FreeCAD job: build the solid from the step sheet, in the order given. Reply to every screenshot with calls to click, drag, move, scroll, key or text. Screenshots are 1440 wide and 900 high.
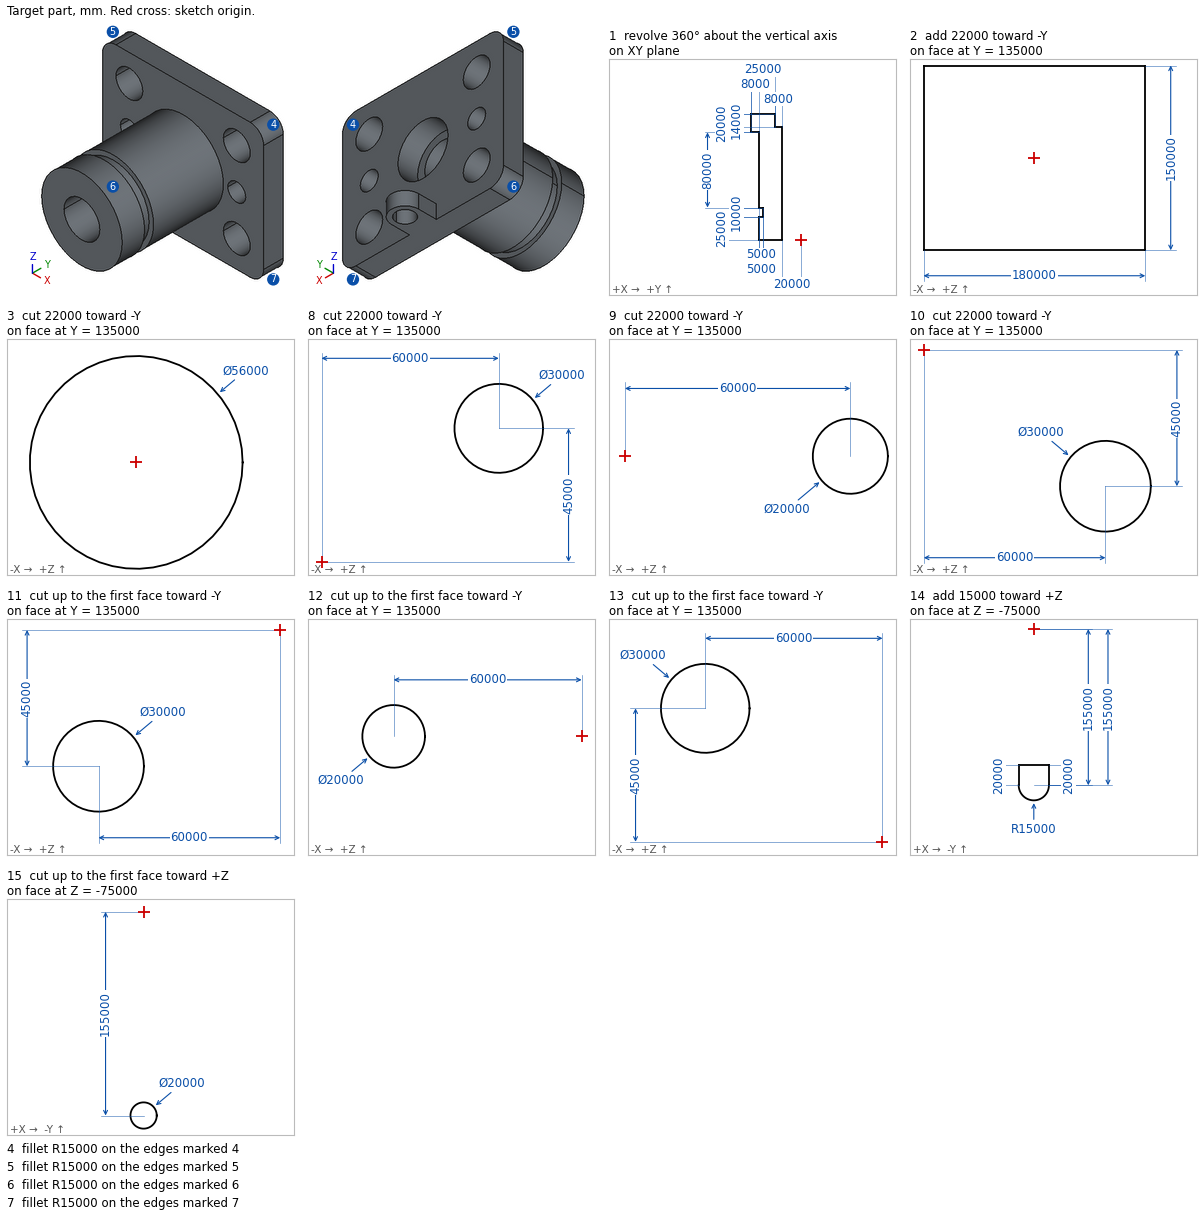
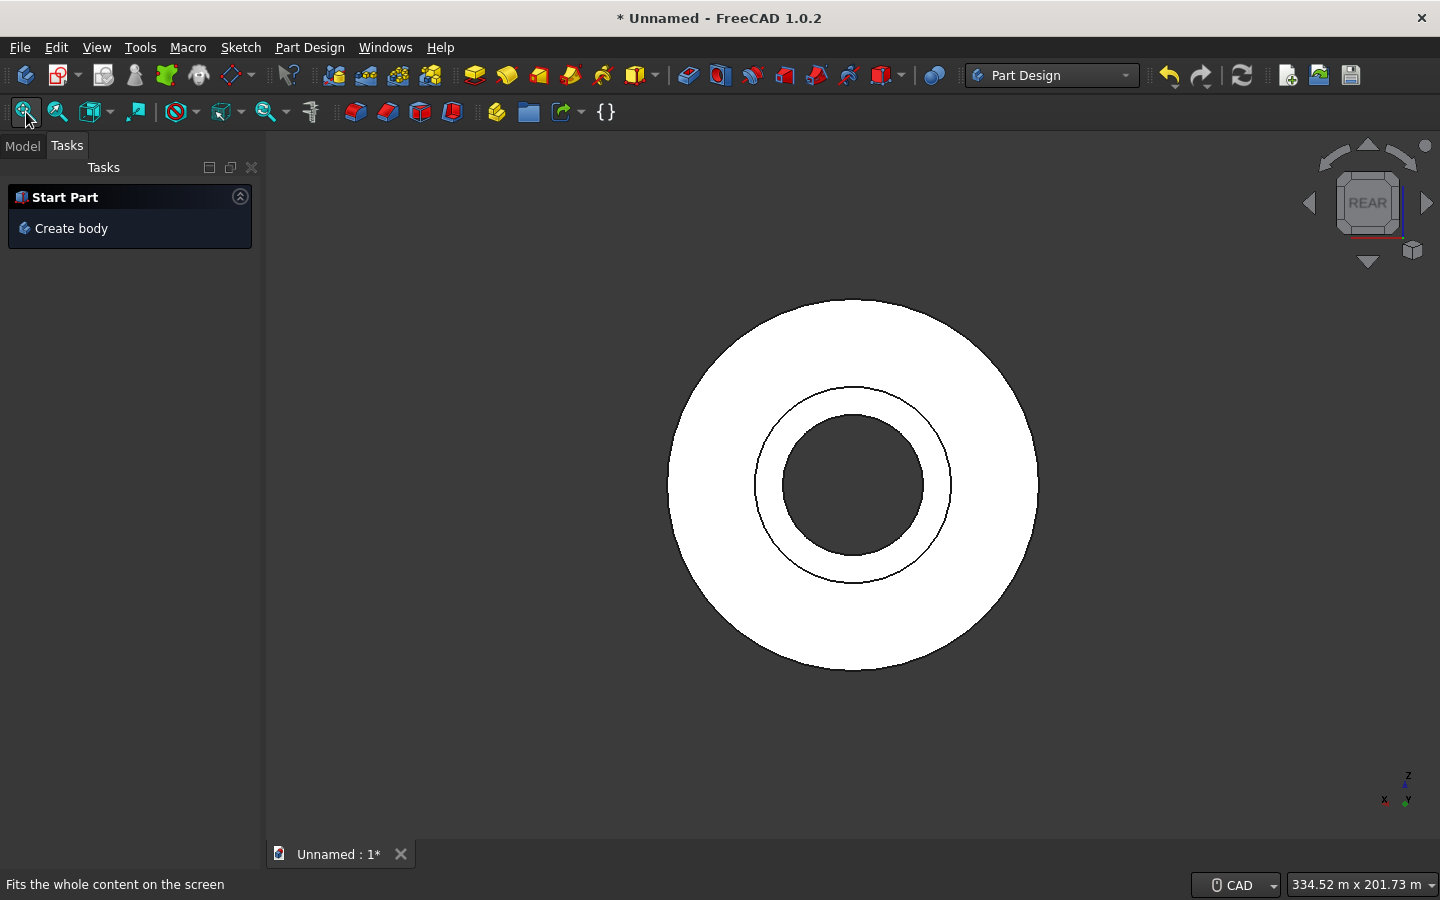
click(747, 590)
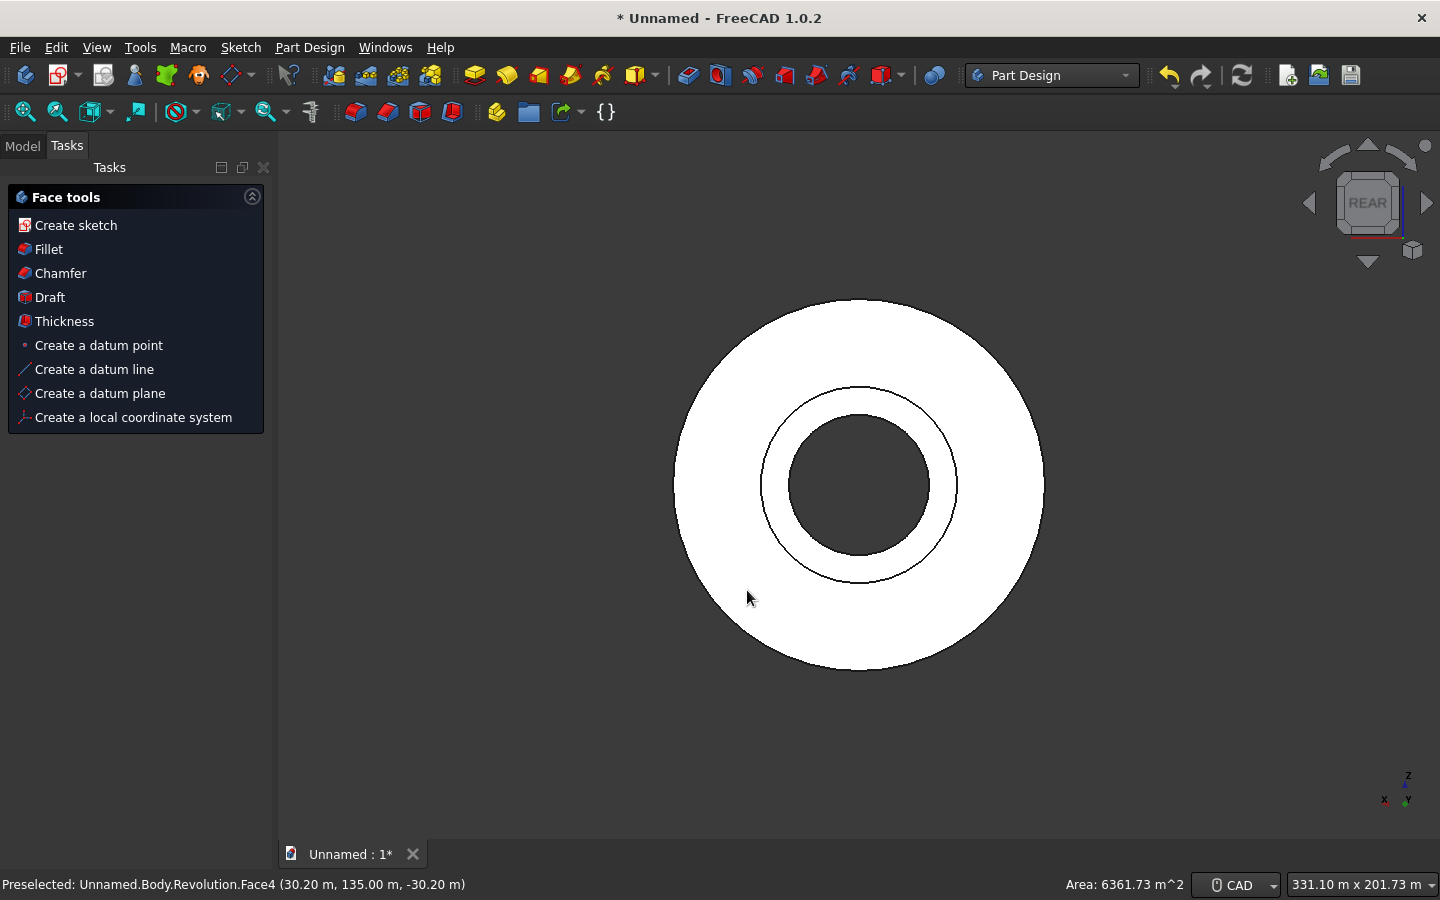
click(58, 76)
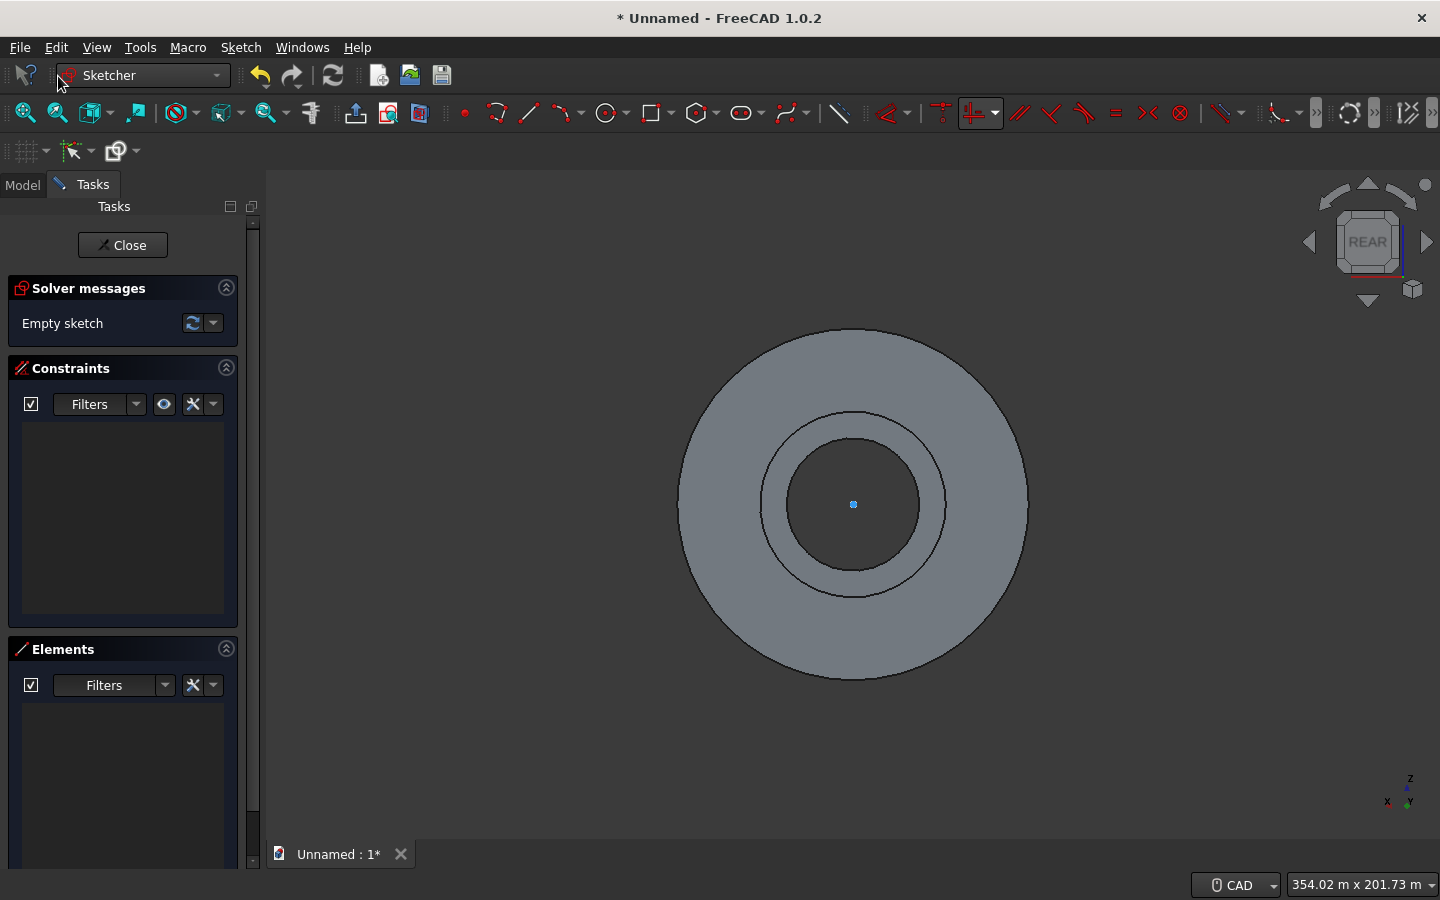
click(674, 114)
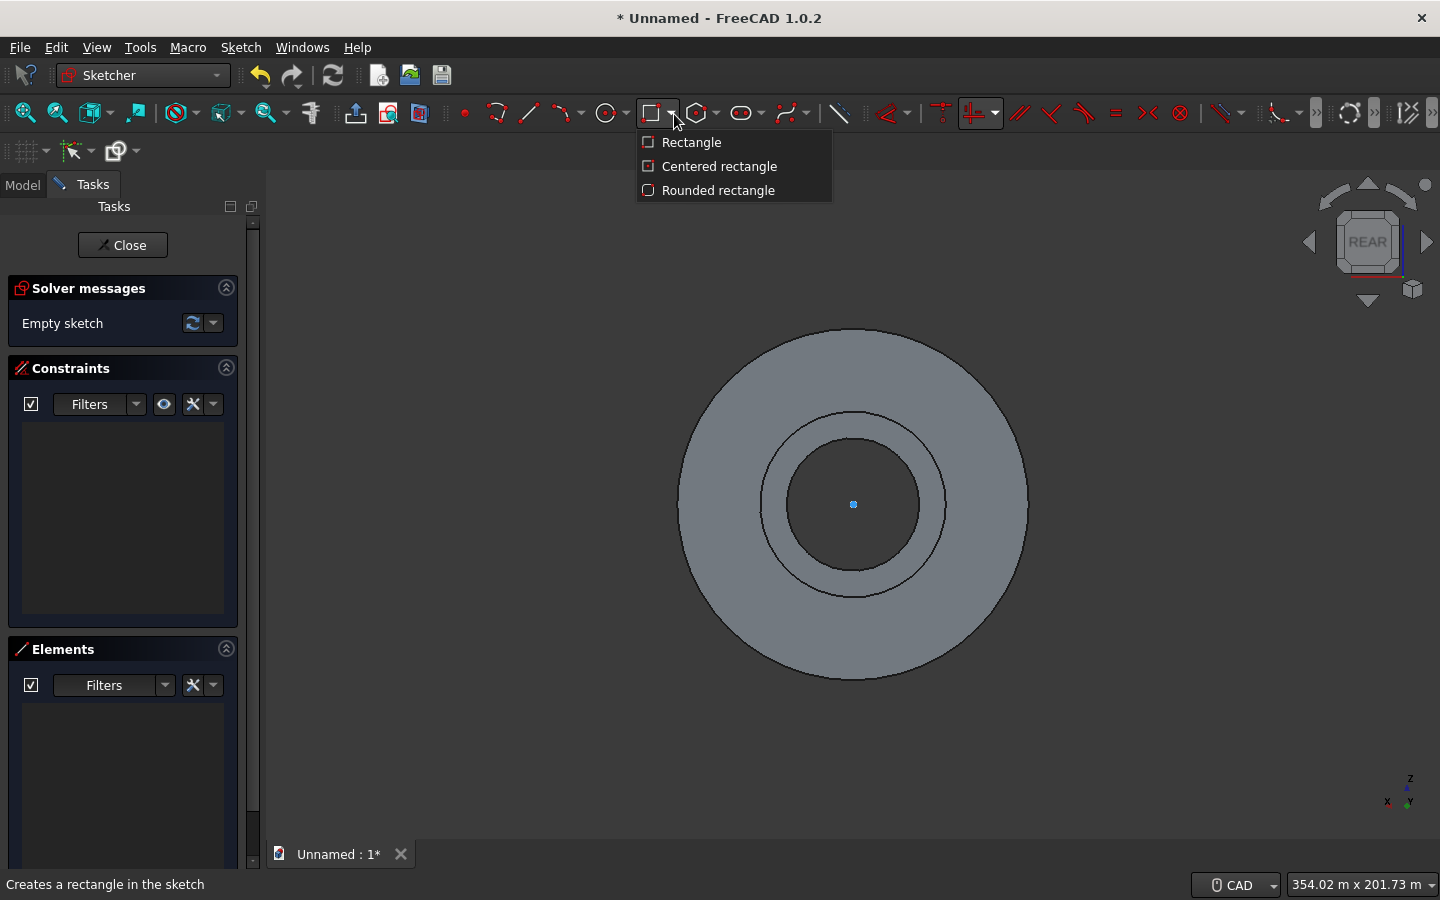
click(734, 166)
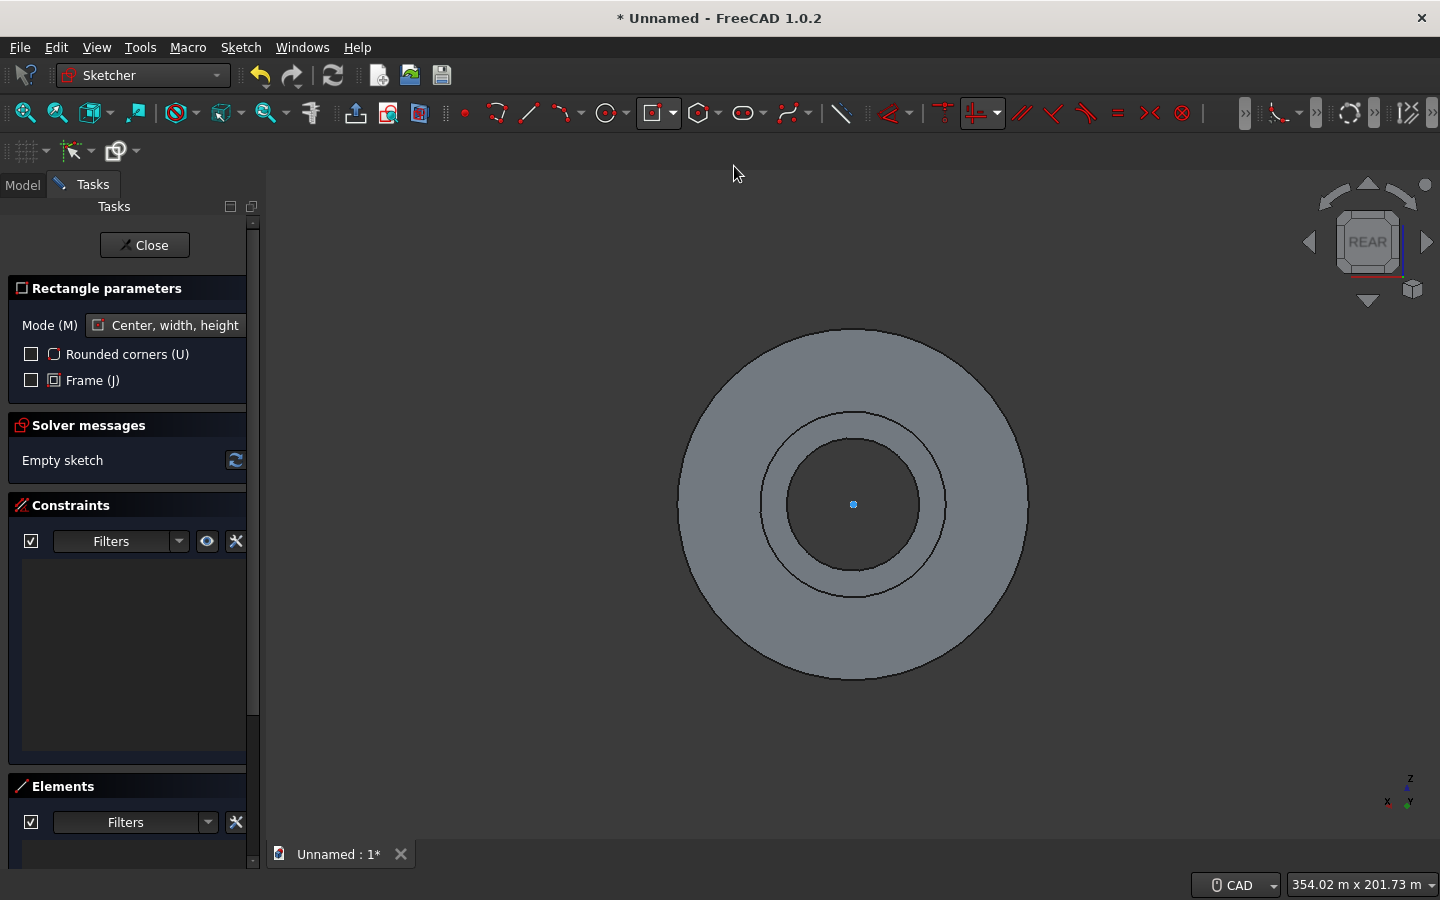
click(853, 505)
click(1151, 256)
key(Escape)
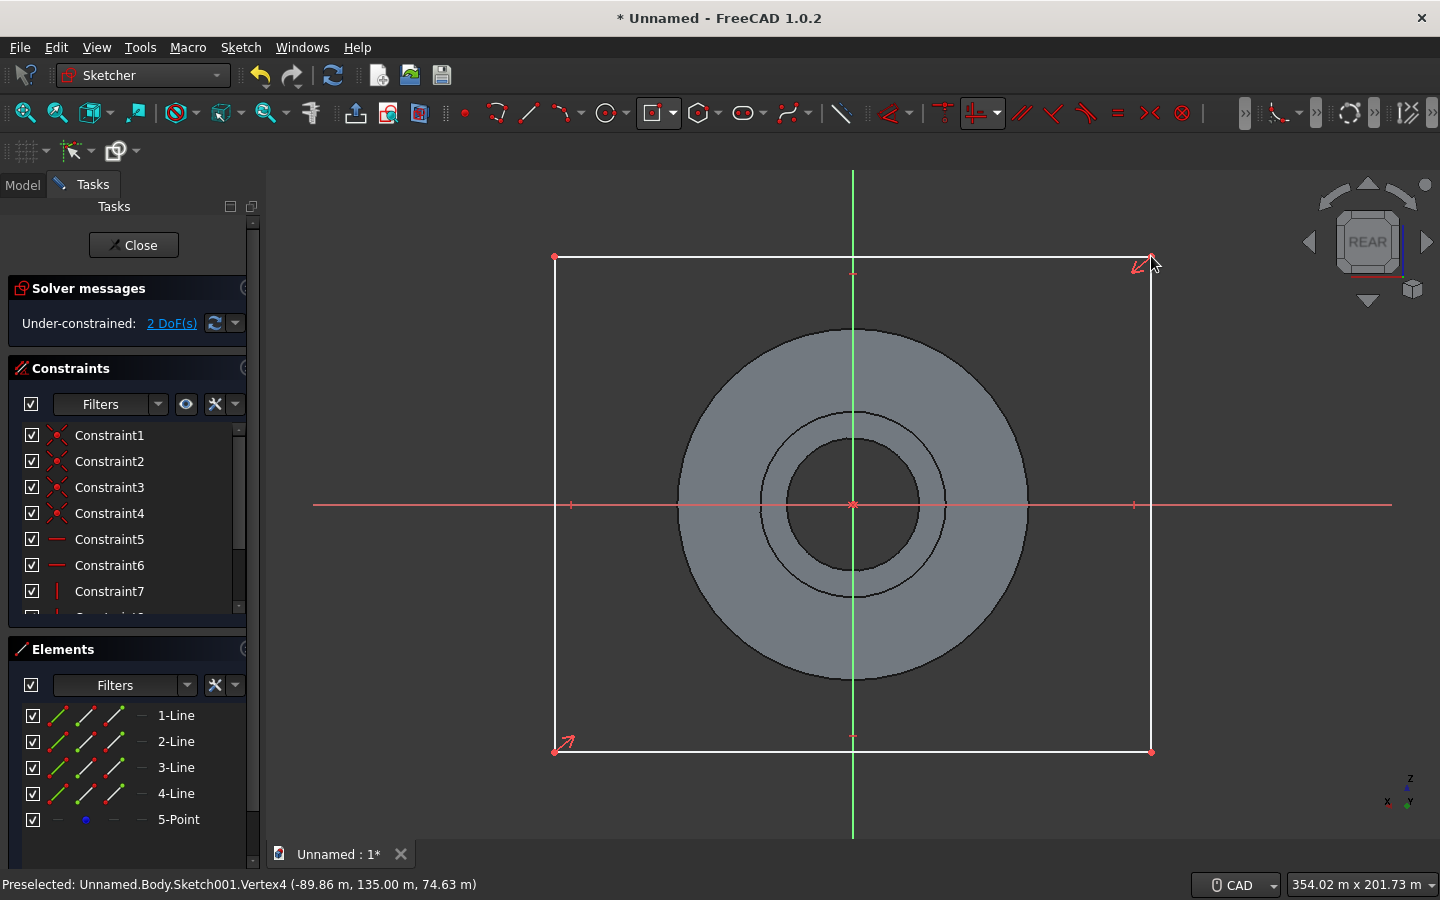
key(d)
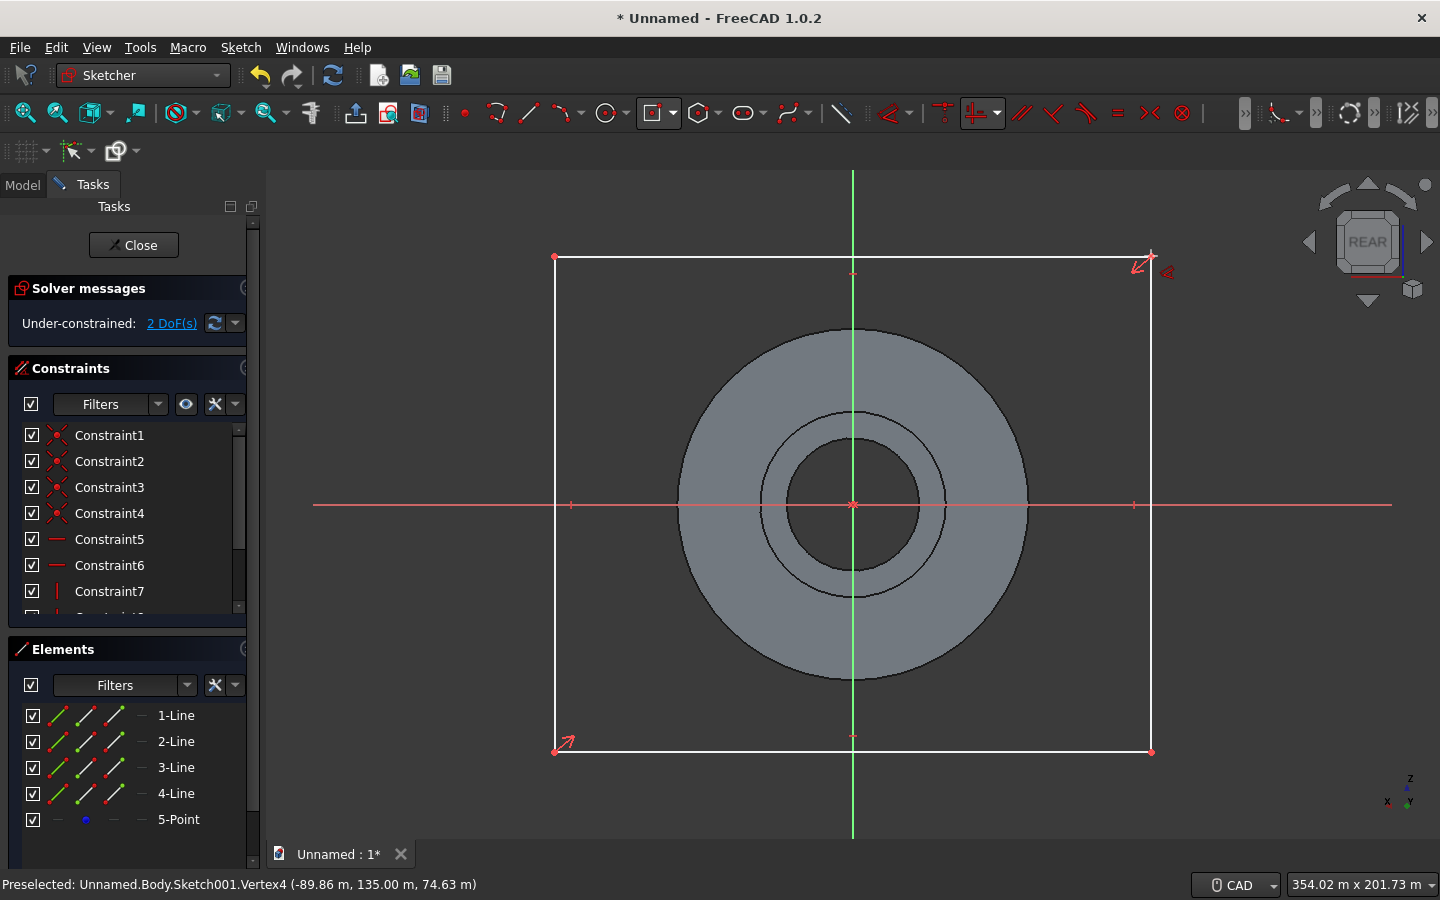
click(734, 752)
click(716, 786)